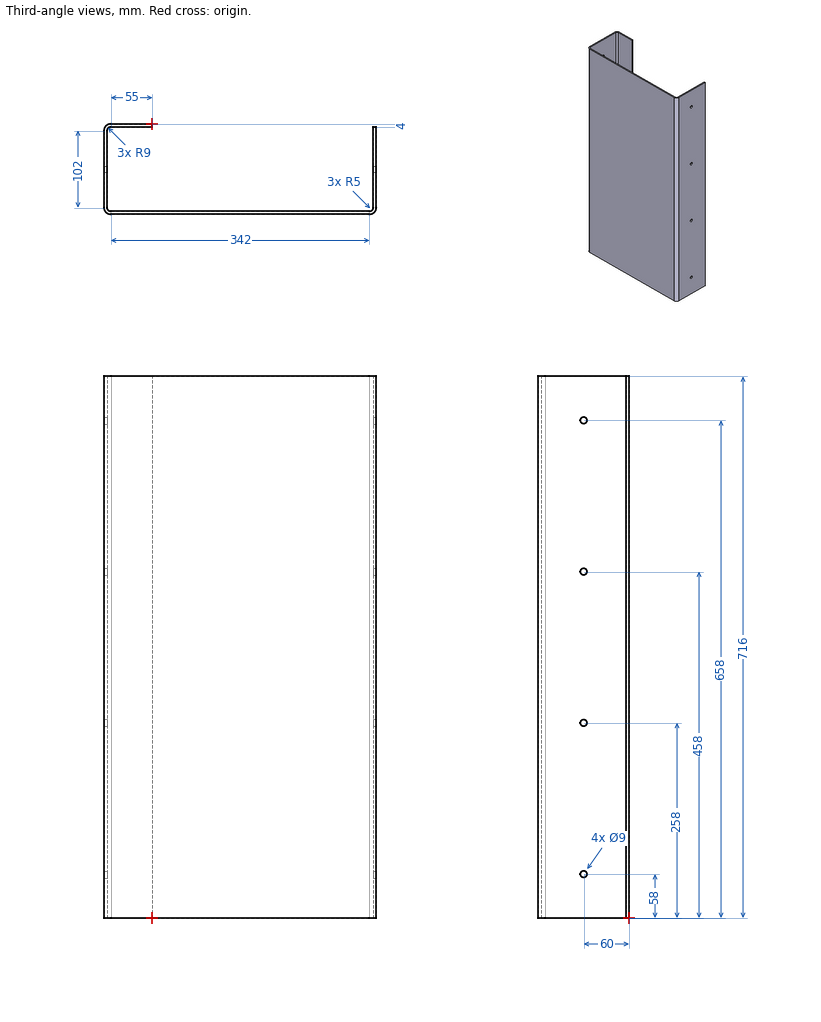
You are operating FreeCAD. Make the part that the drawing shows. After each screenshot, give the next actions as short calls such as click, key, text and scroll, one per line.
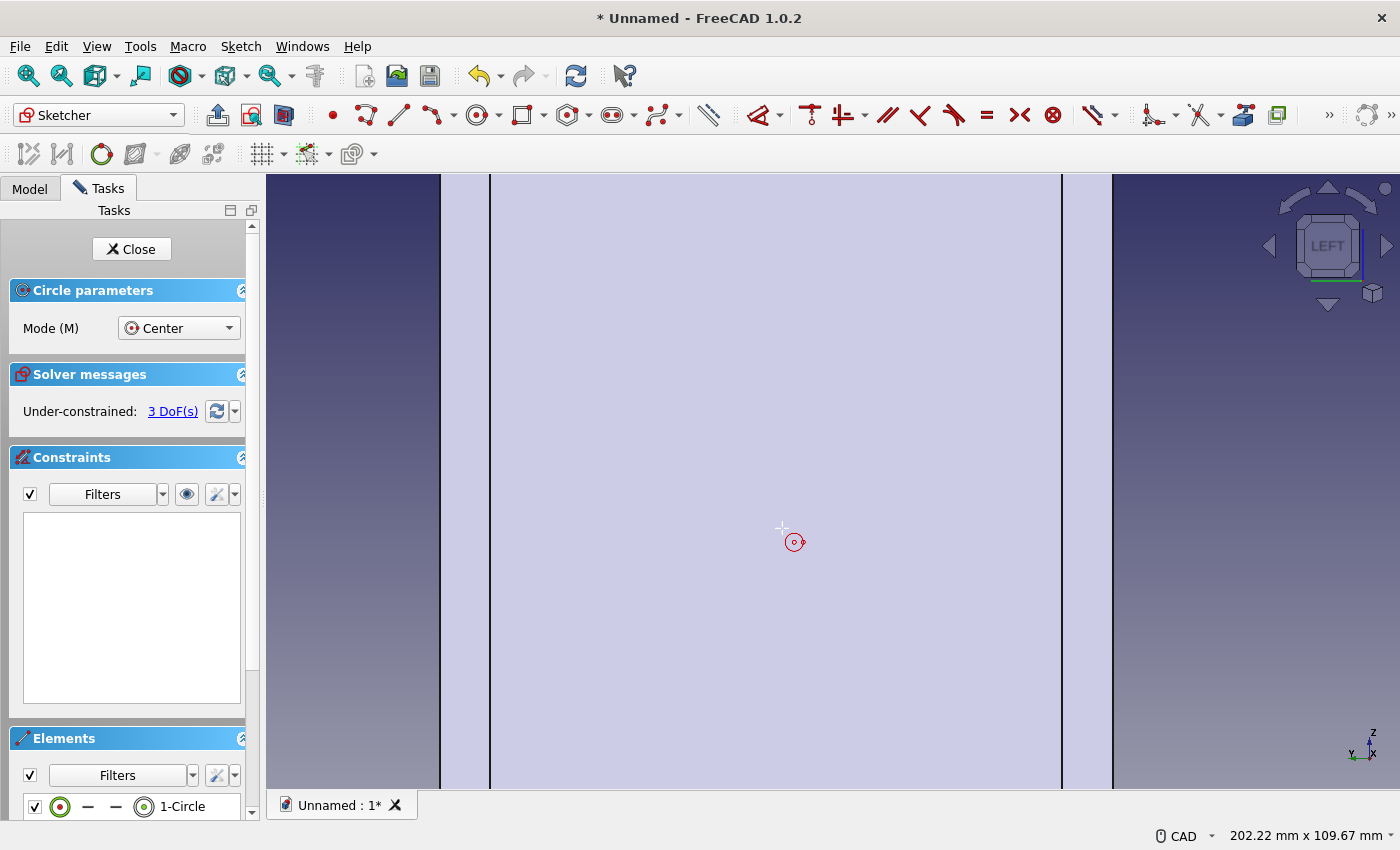
scroll(782, 527, down, 11)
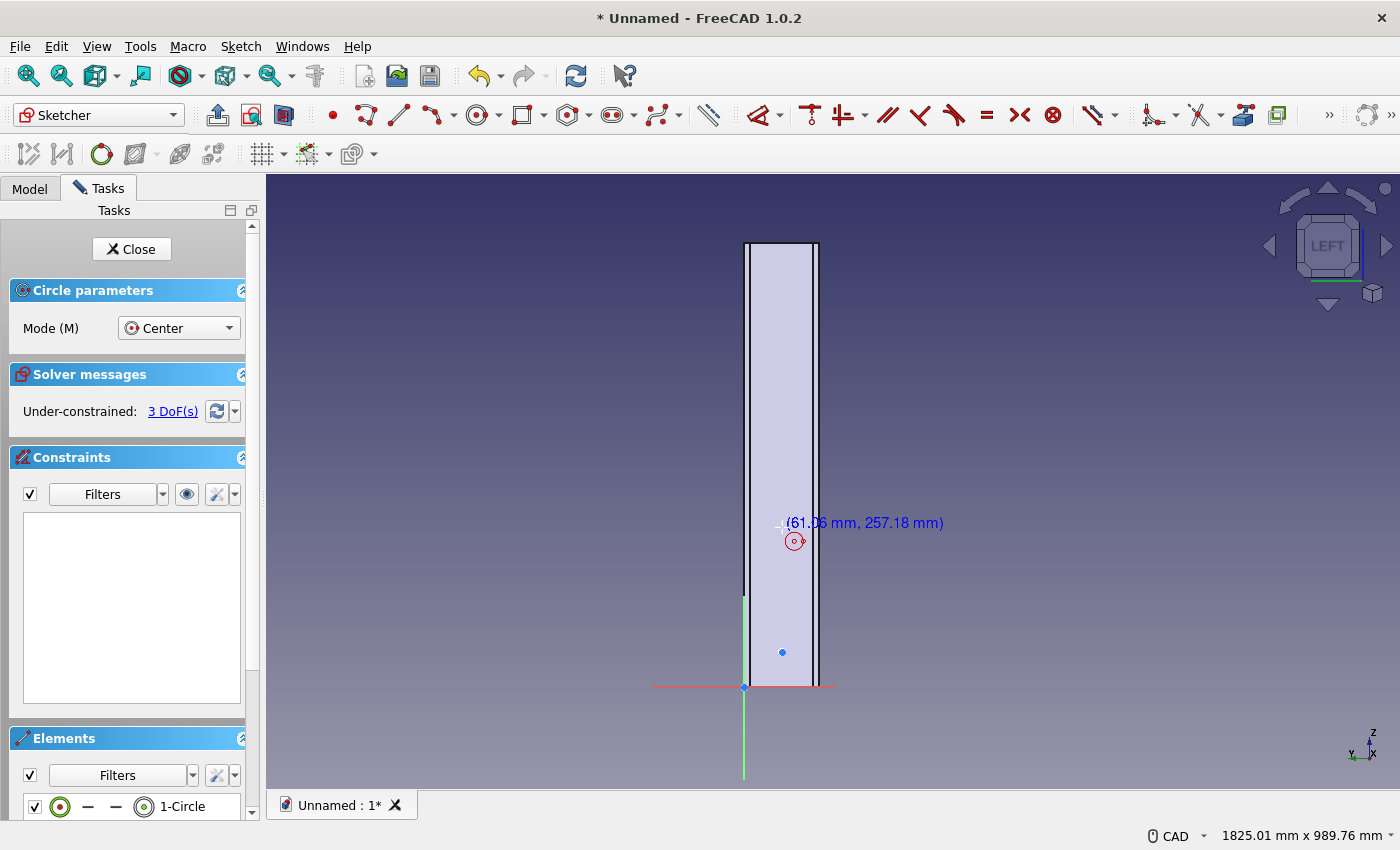
click(782, 527)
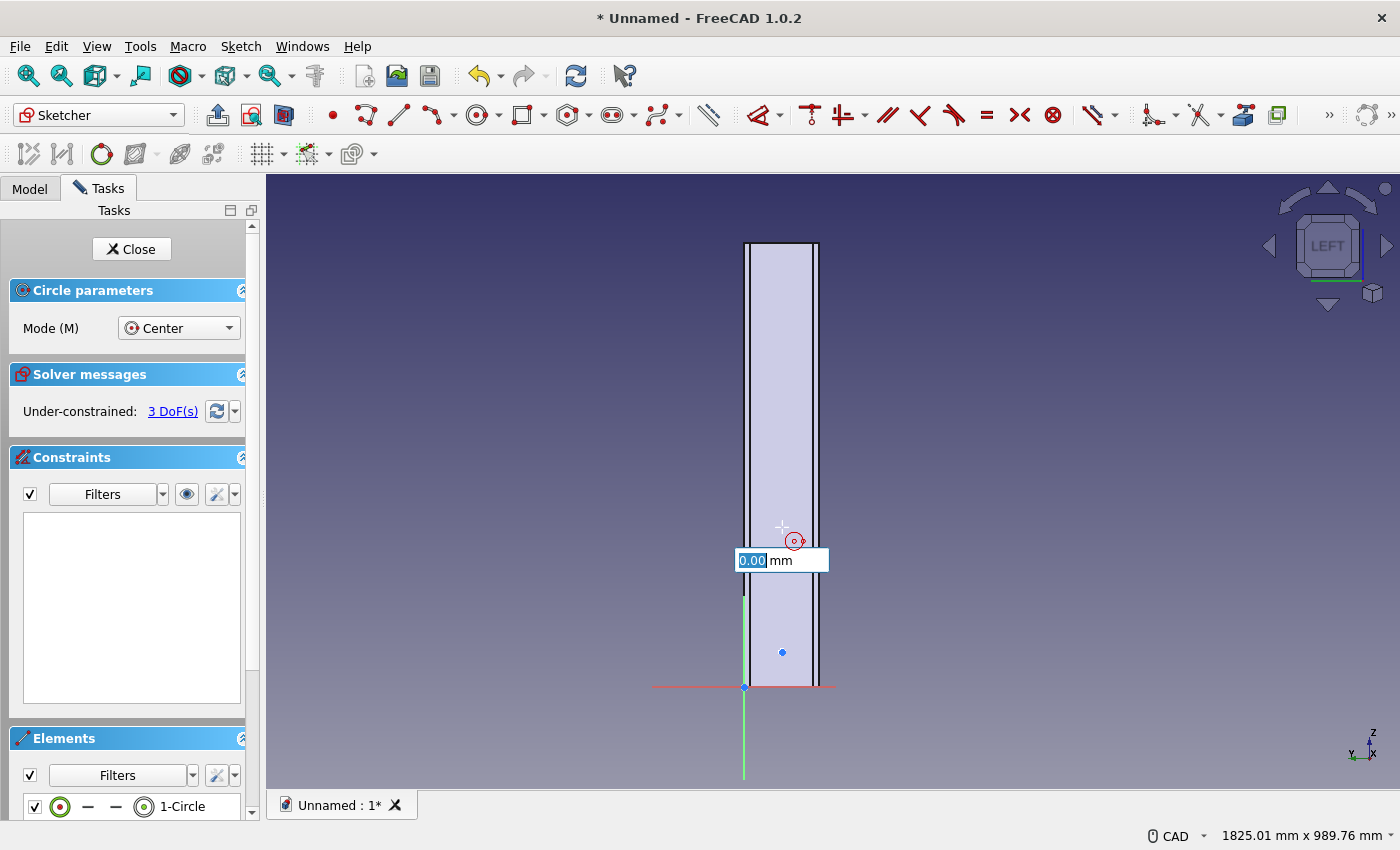
scroll(784, 525, up, 9)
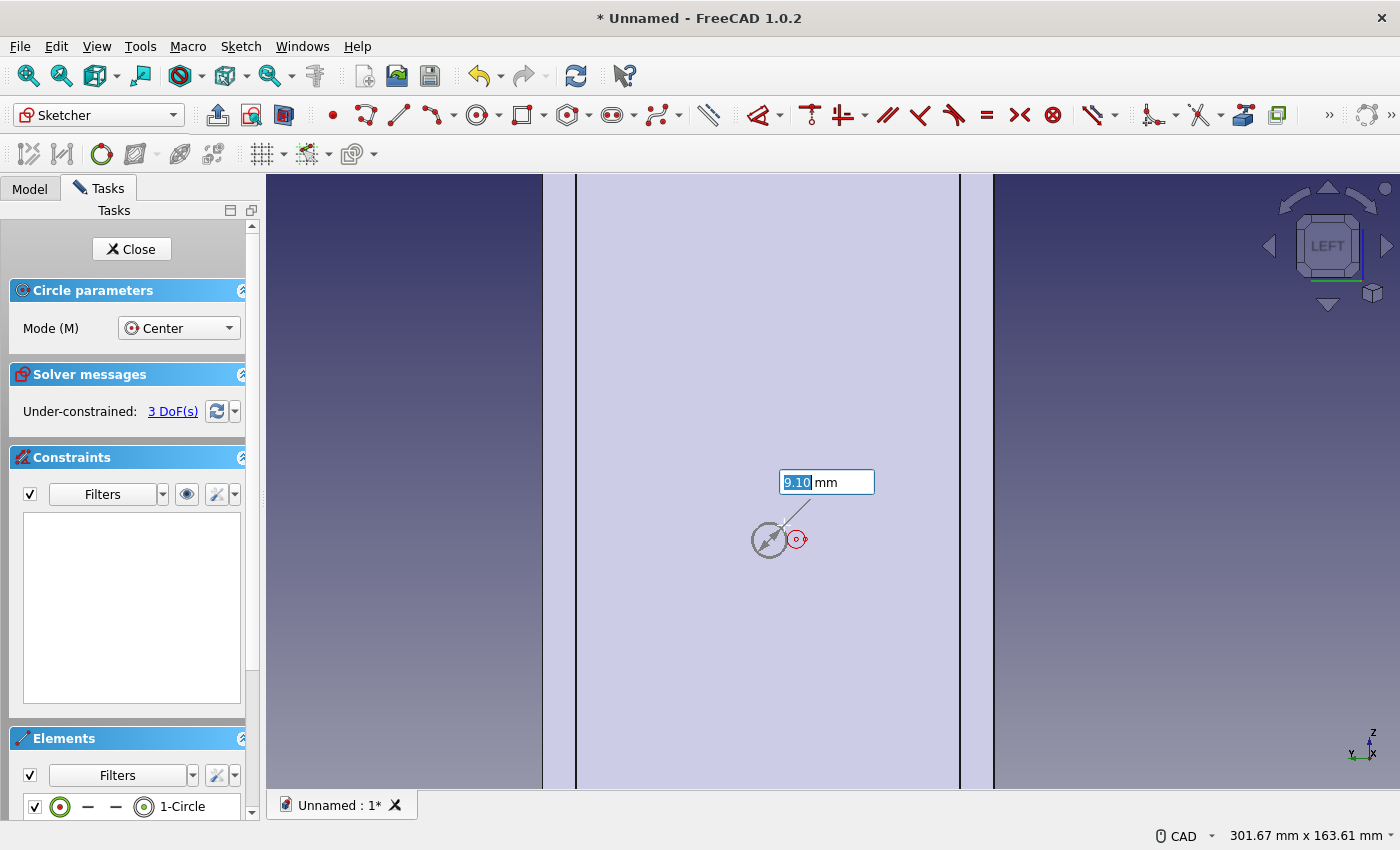
click(780, 523)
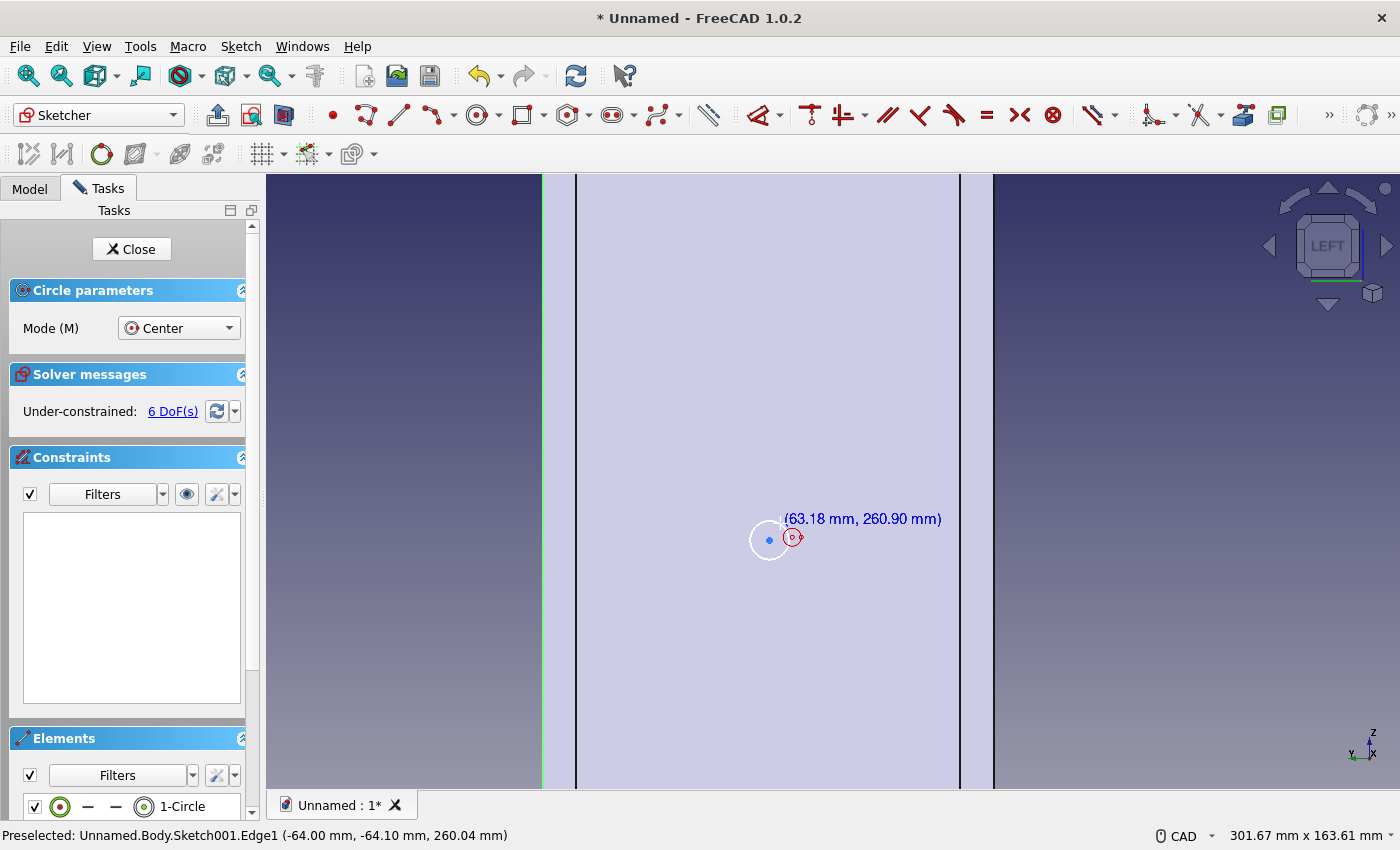
scroll(784, 525, down, 9)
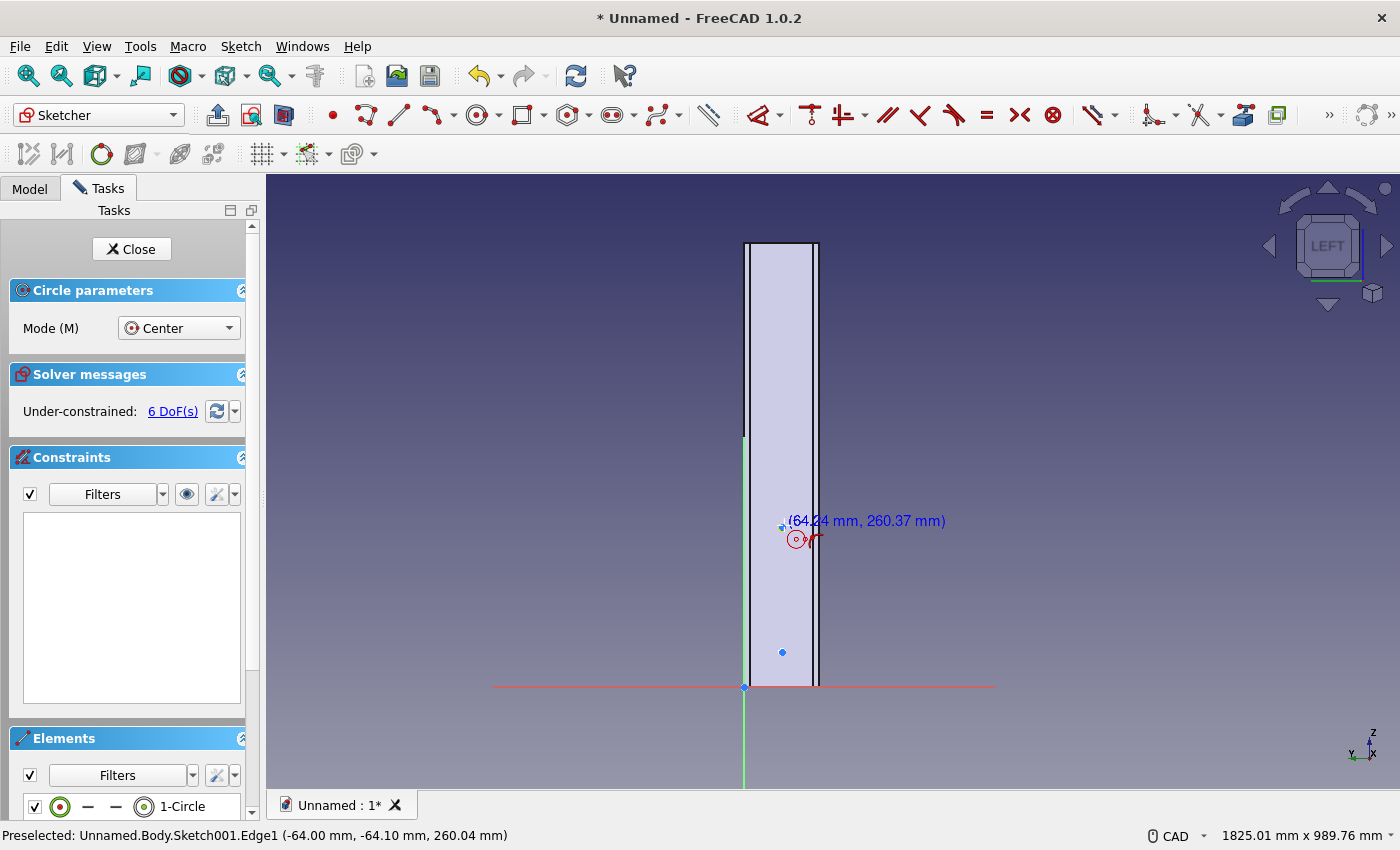
scroll(782, 403, up, 11)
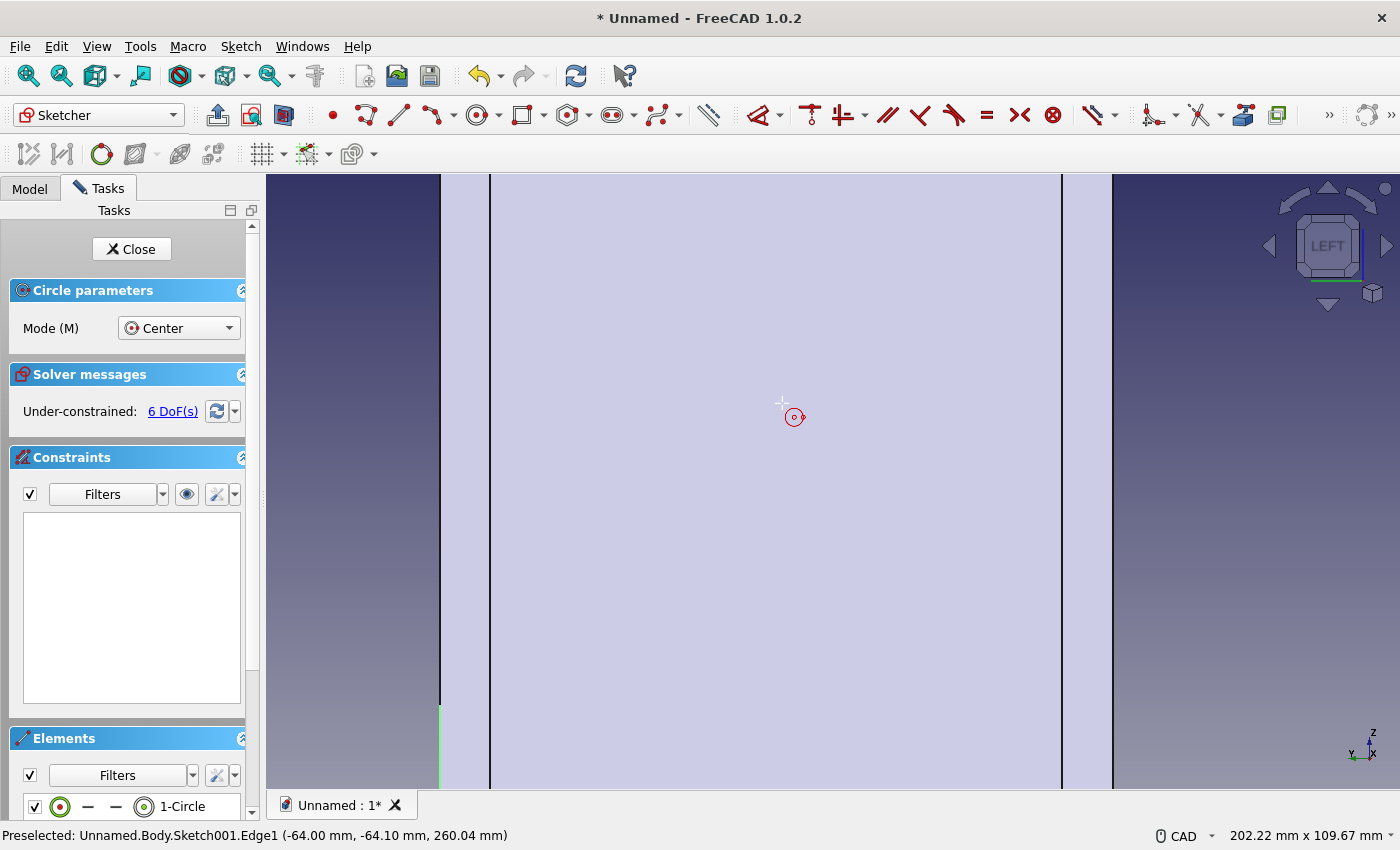
scroll(782, 403, down, 11)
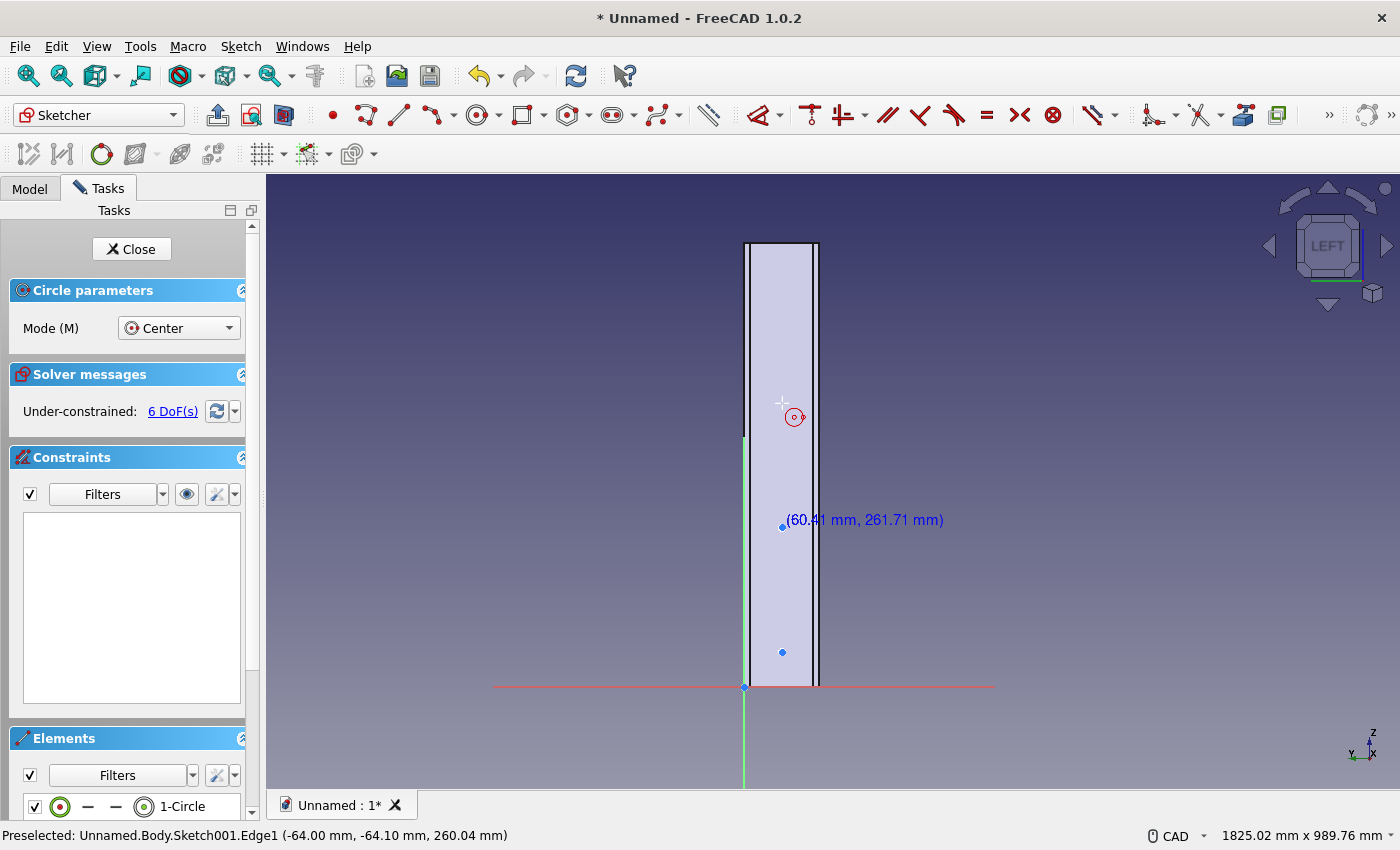
click(782, 403)